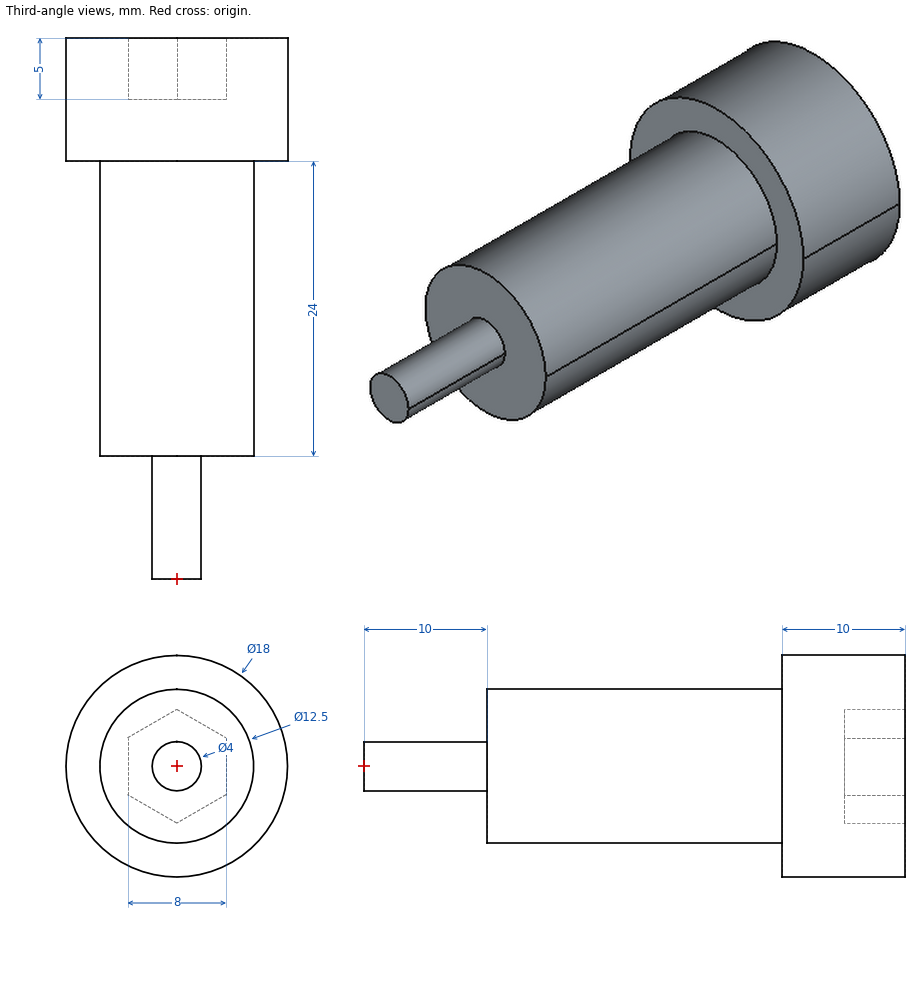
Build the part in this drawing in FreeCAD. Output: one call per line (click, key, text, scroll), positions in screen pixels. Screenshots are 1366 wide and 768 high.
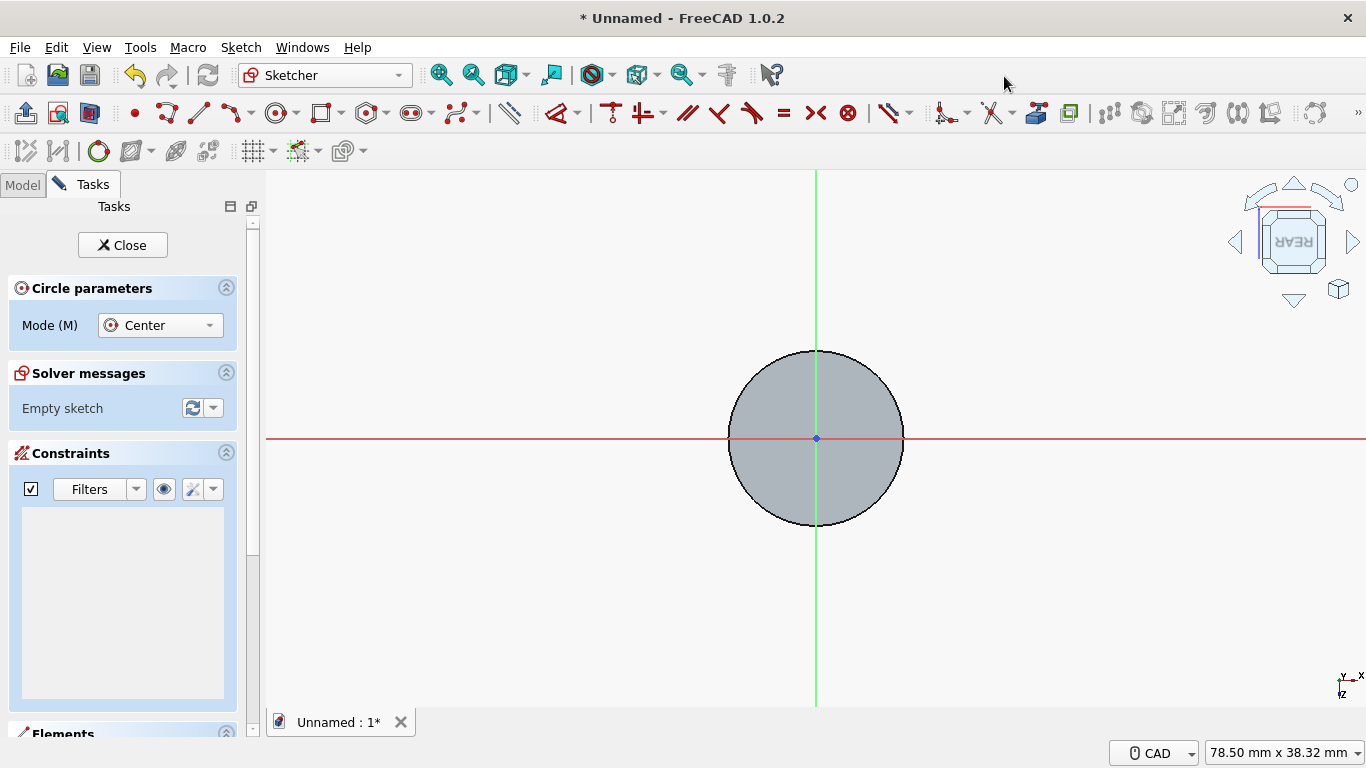
click(816, 438)
move(905, 349)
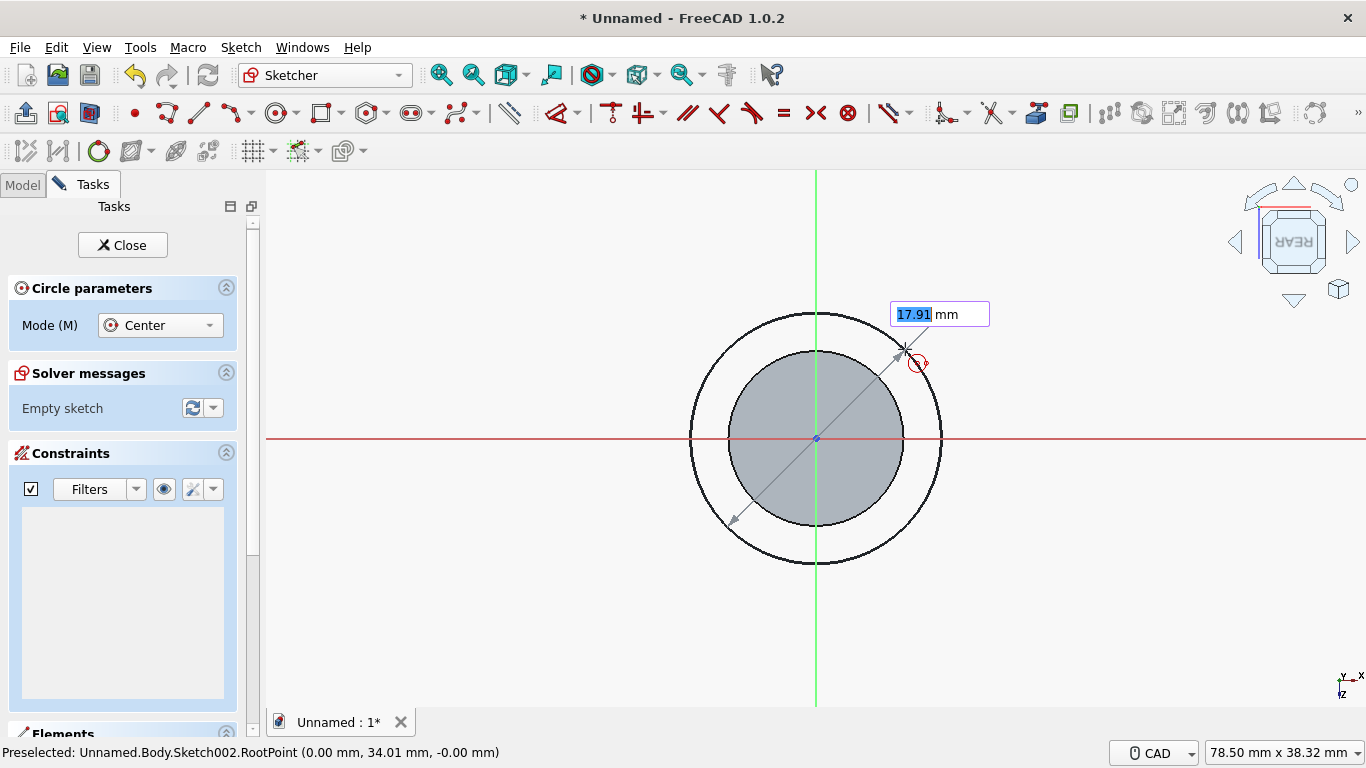
text(18)
key(Return)
key(Escape)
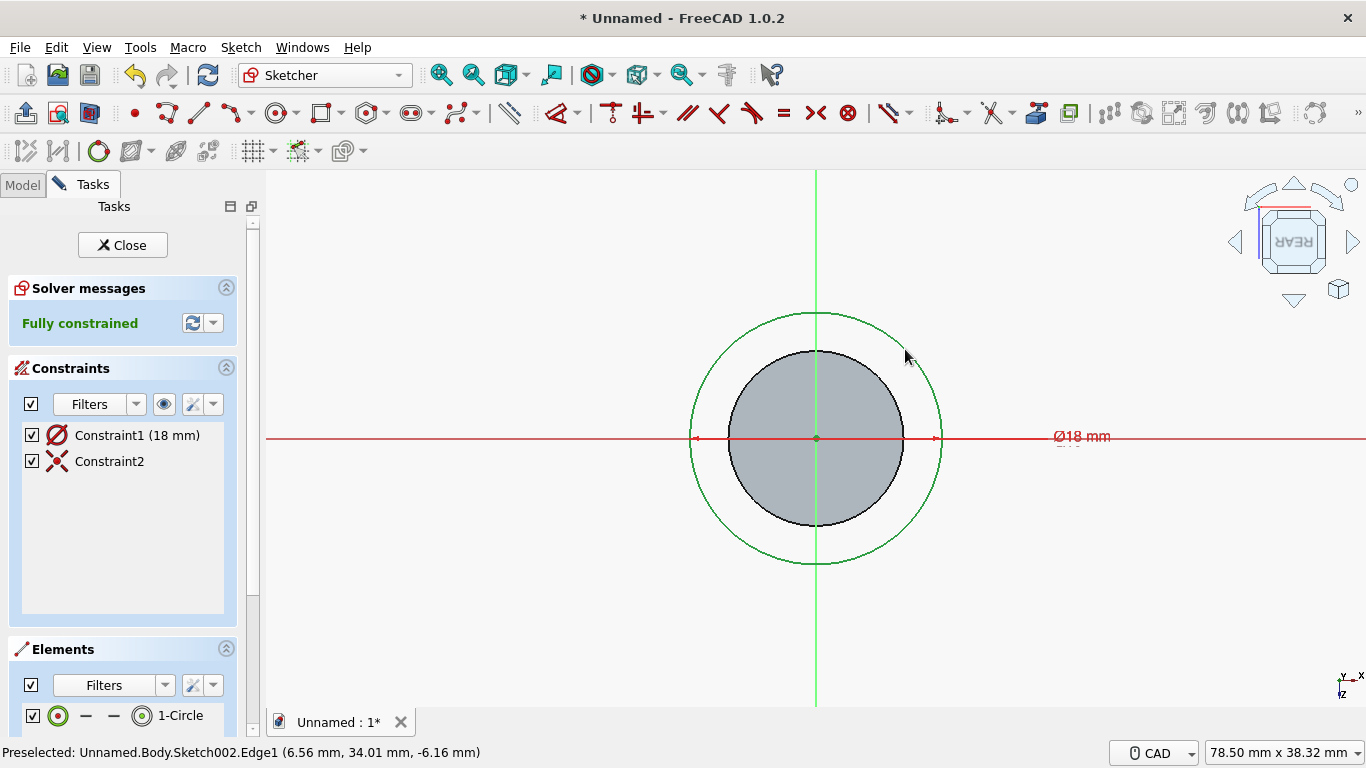
click(123, 245)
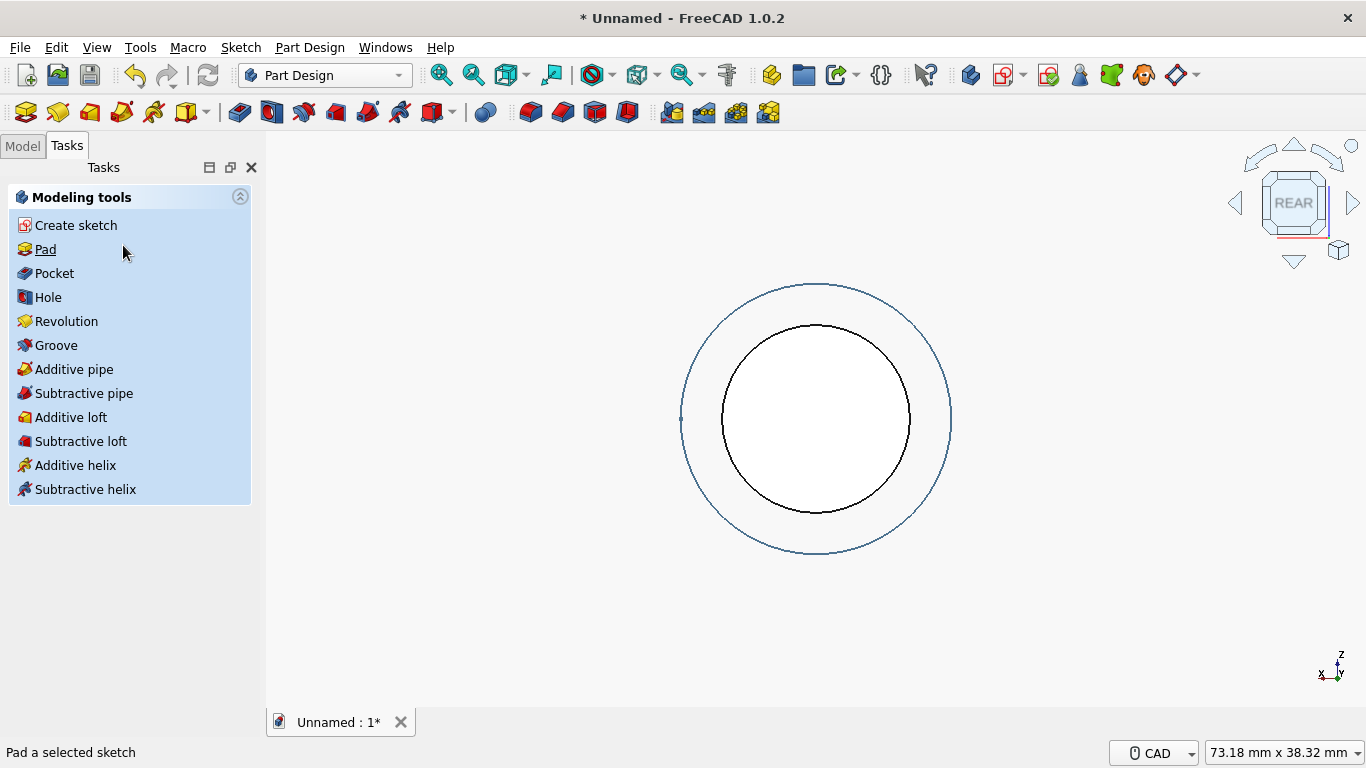
click(26, 112)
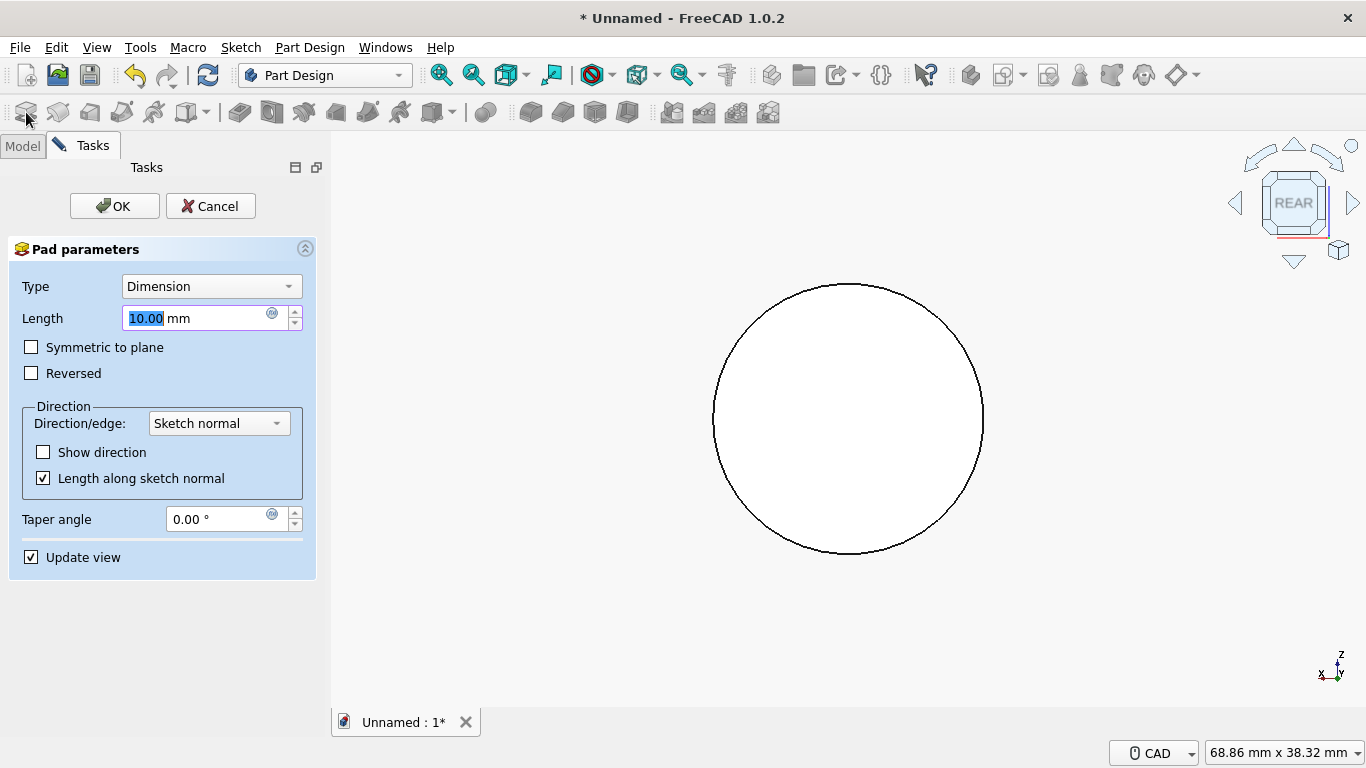
text(10)
key(Tab)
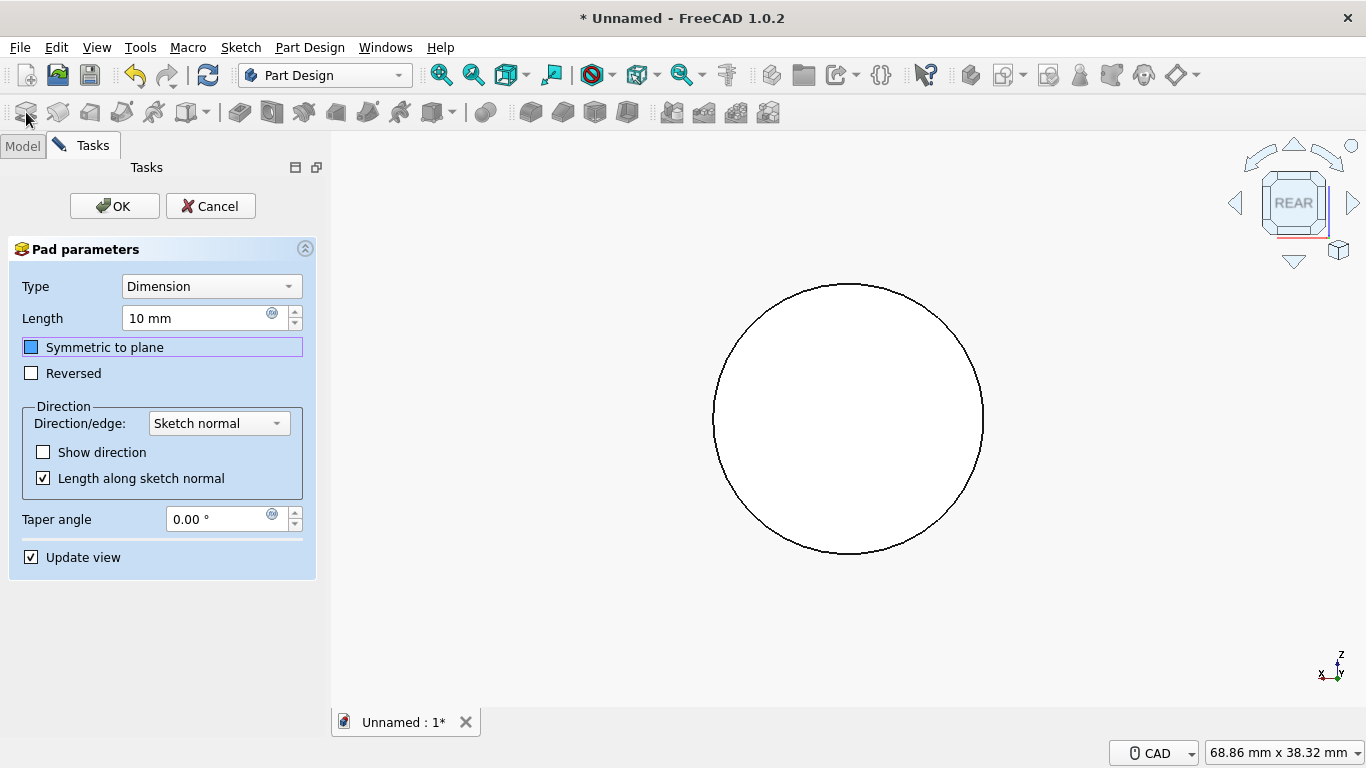
click(115, 206)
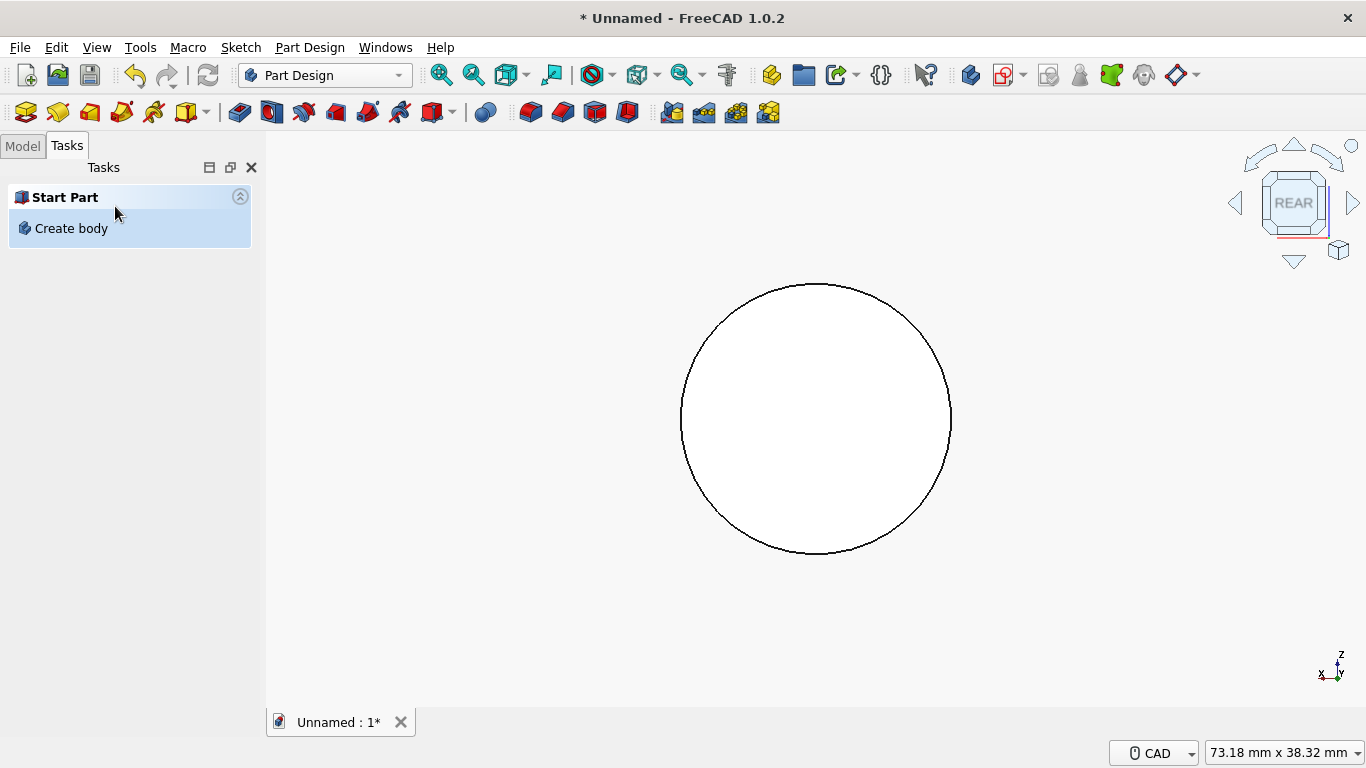
click(816, 418)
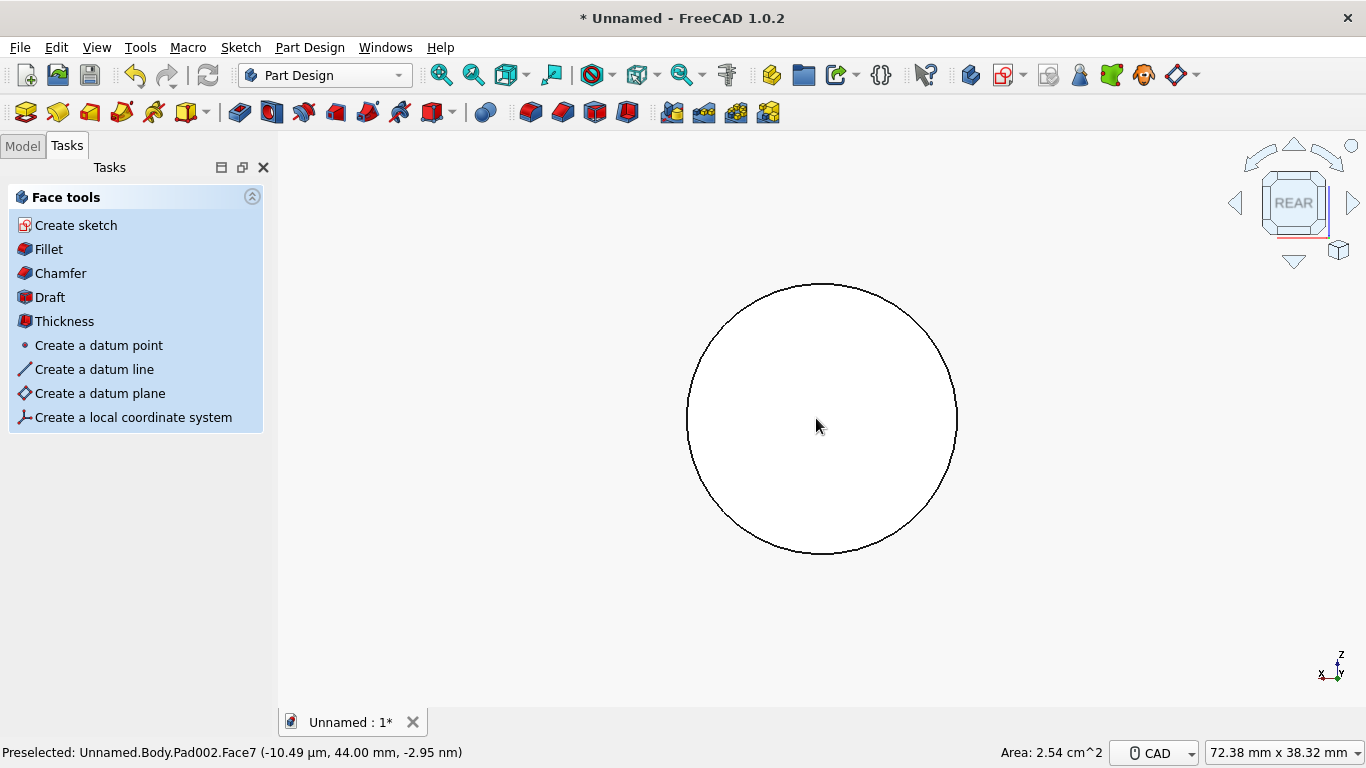
click(1004, 76)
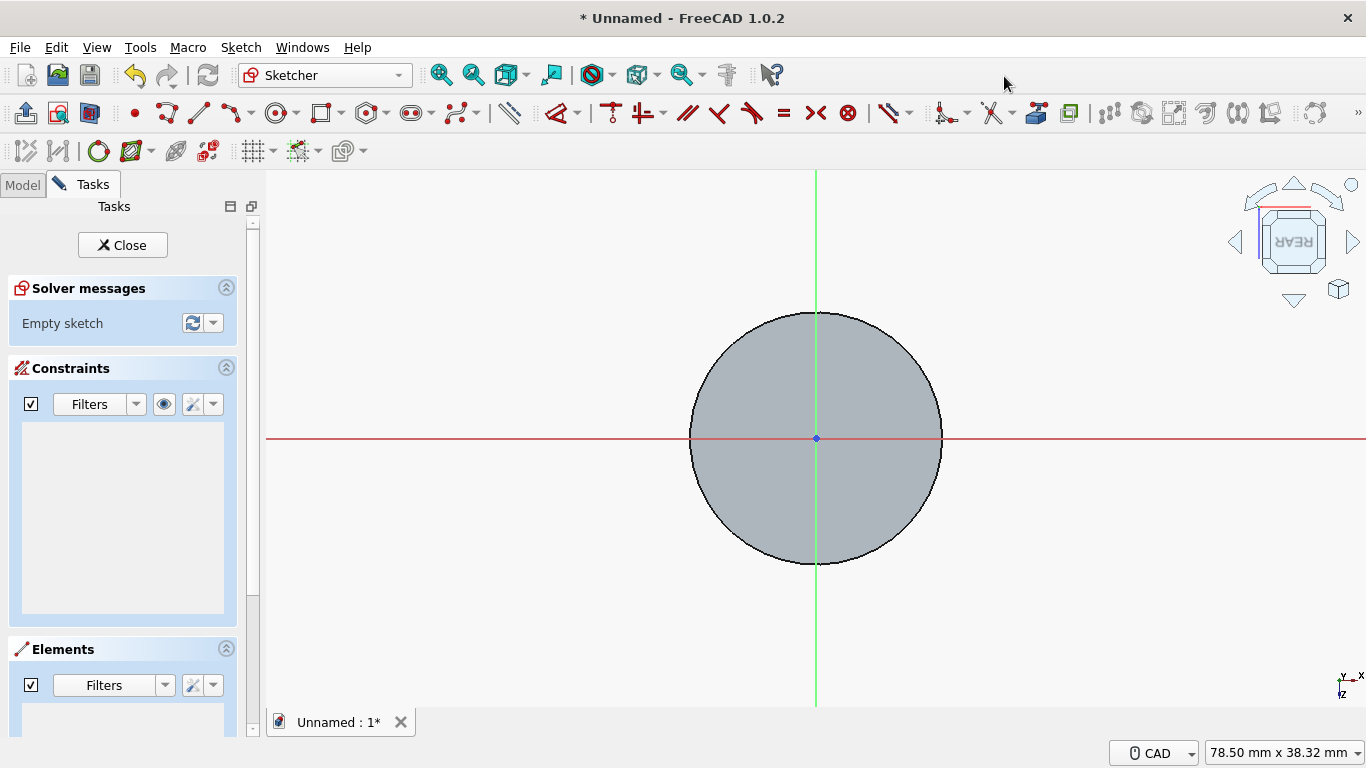
scroll(856, 438, up, 5)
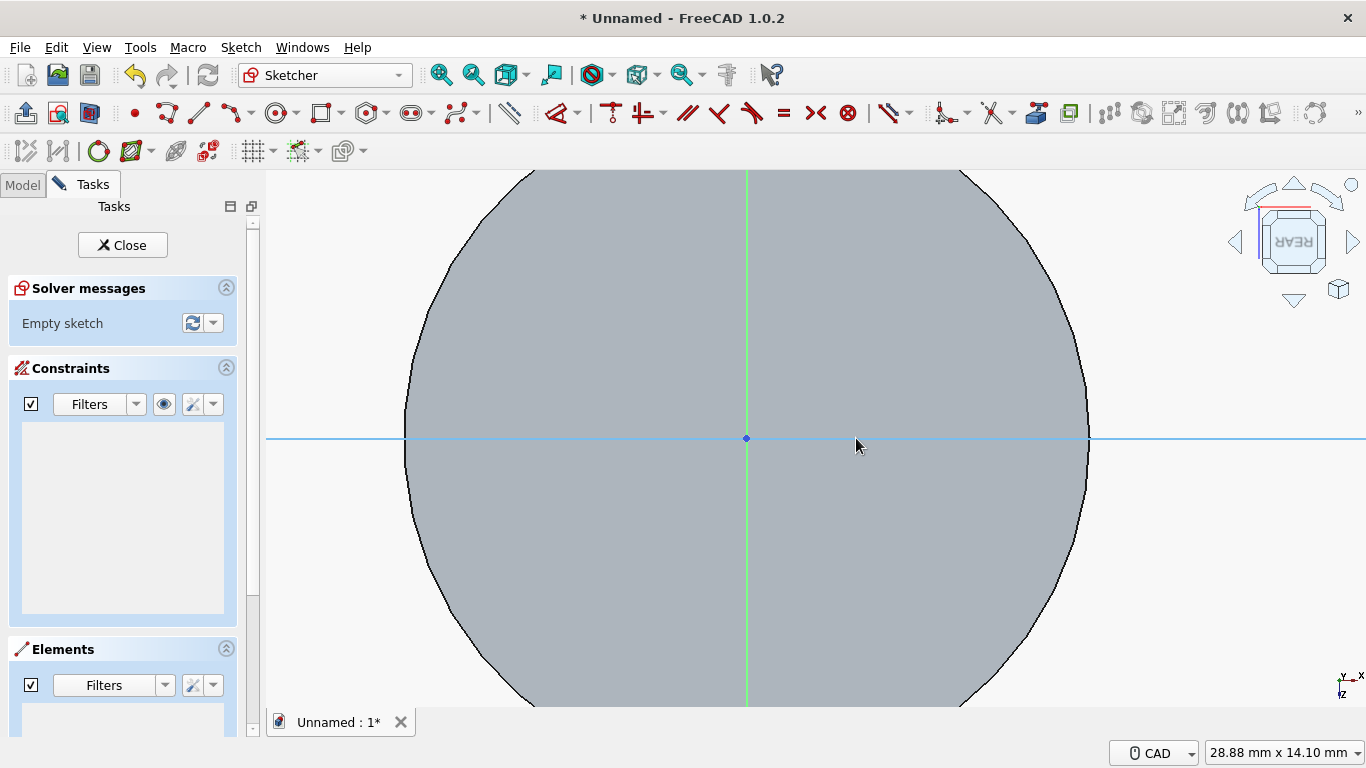
key(g)
key(p)
key(6)